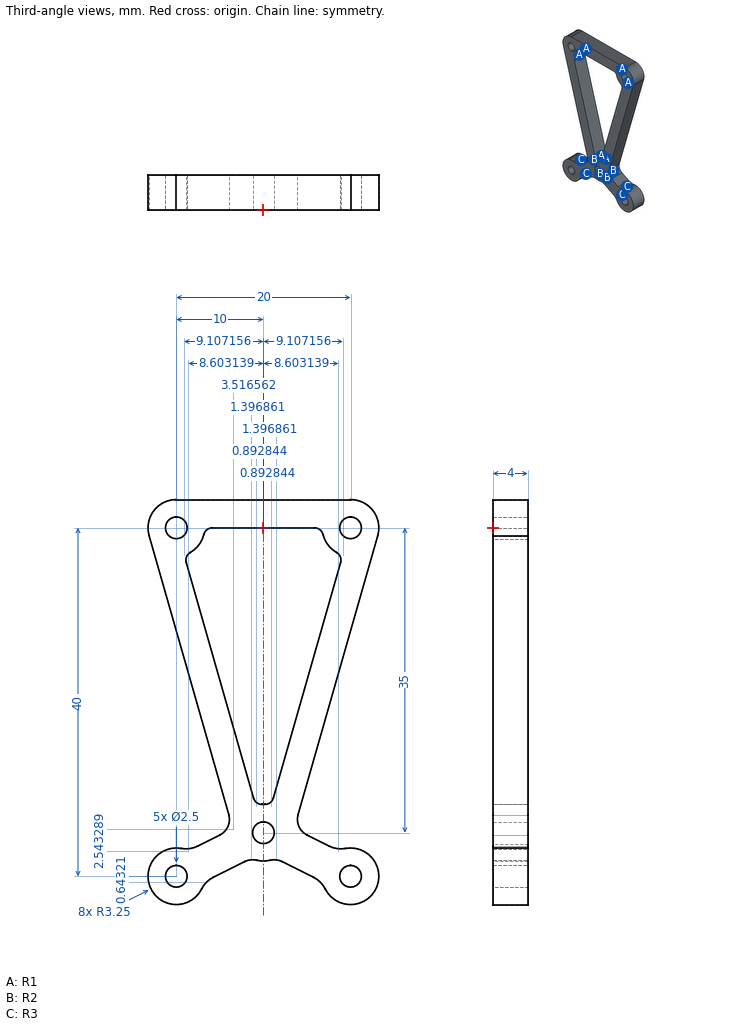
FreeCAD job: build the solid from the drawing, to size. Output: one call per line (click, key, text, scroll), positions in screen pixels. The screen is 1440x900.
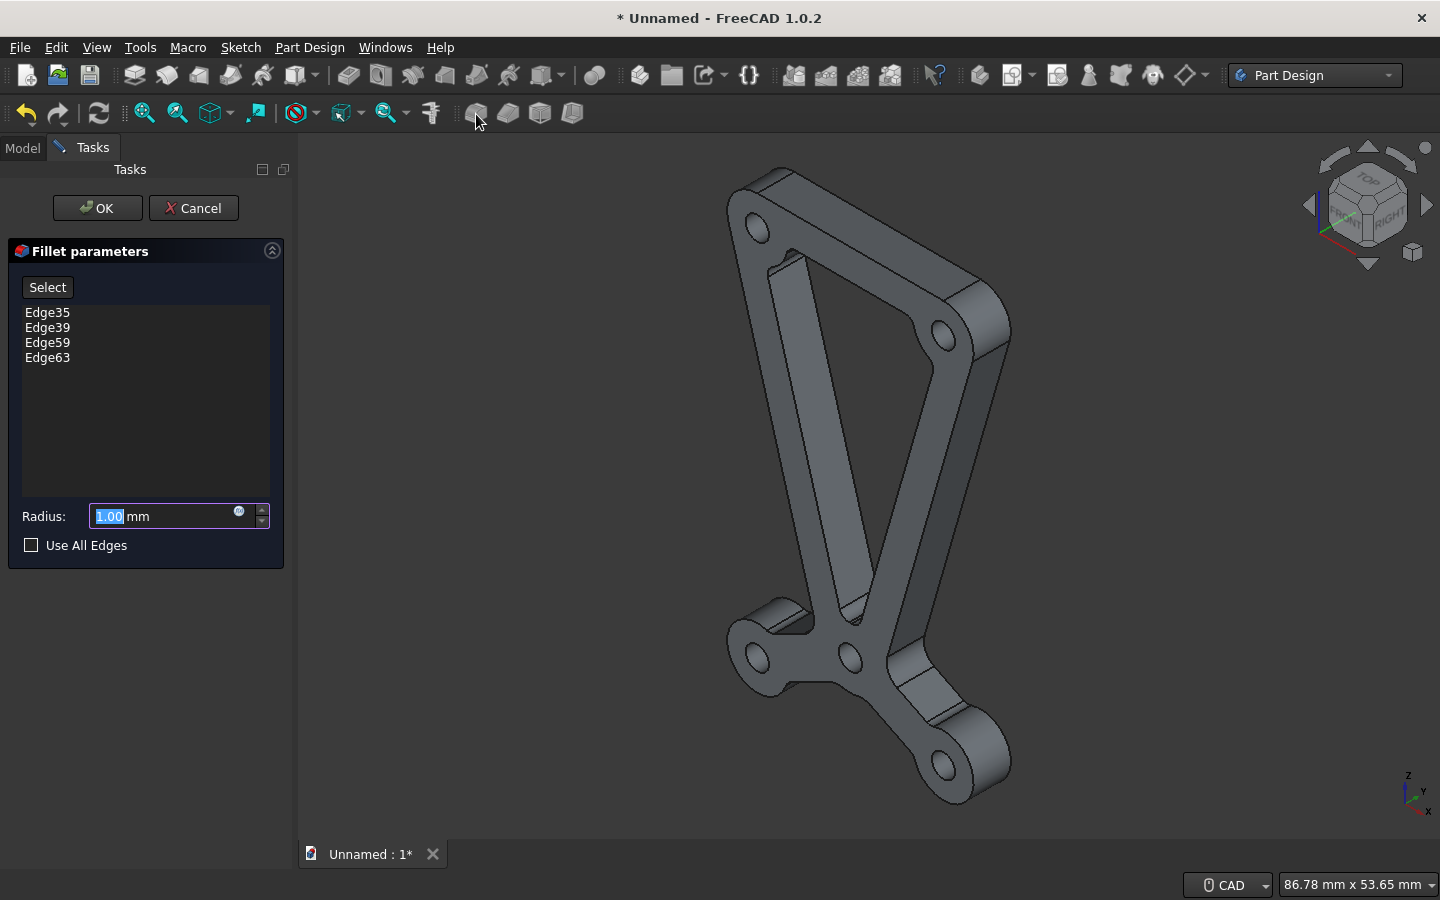
text(3)
key(Tab)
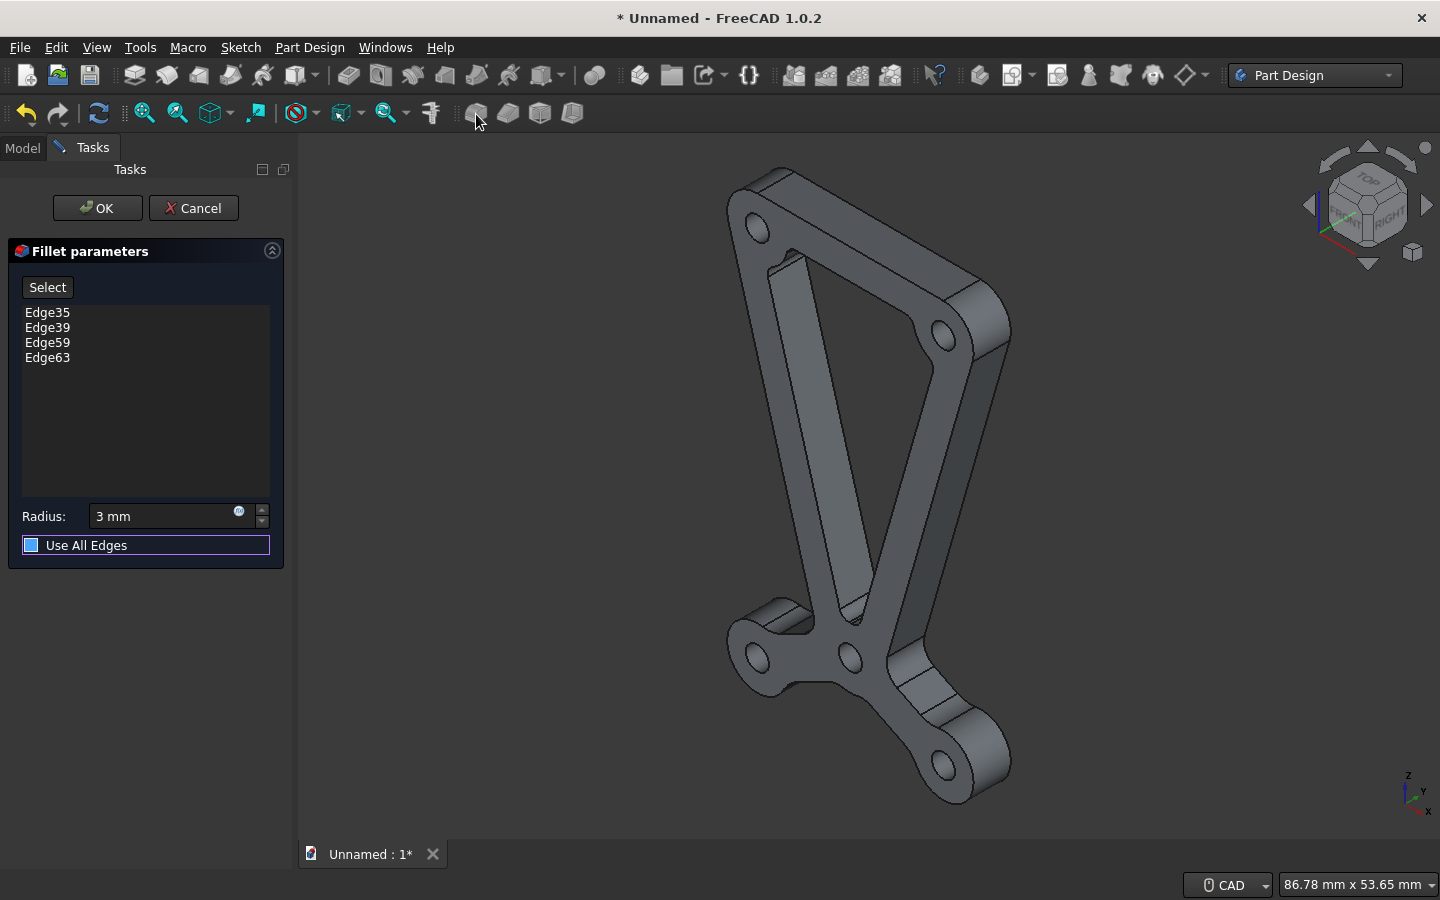
click(98, 208)